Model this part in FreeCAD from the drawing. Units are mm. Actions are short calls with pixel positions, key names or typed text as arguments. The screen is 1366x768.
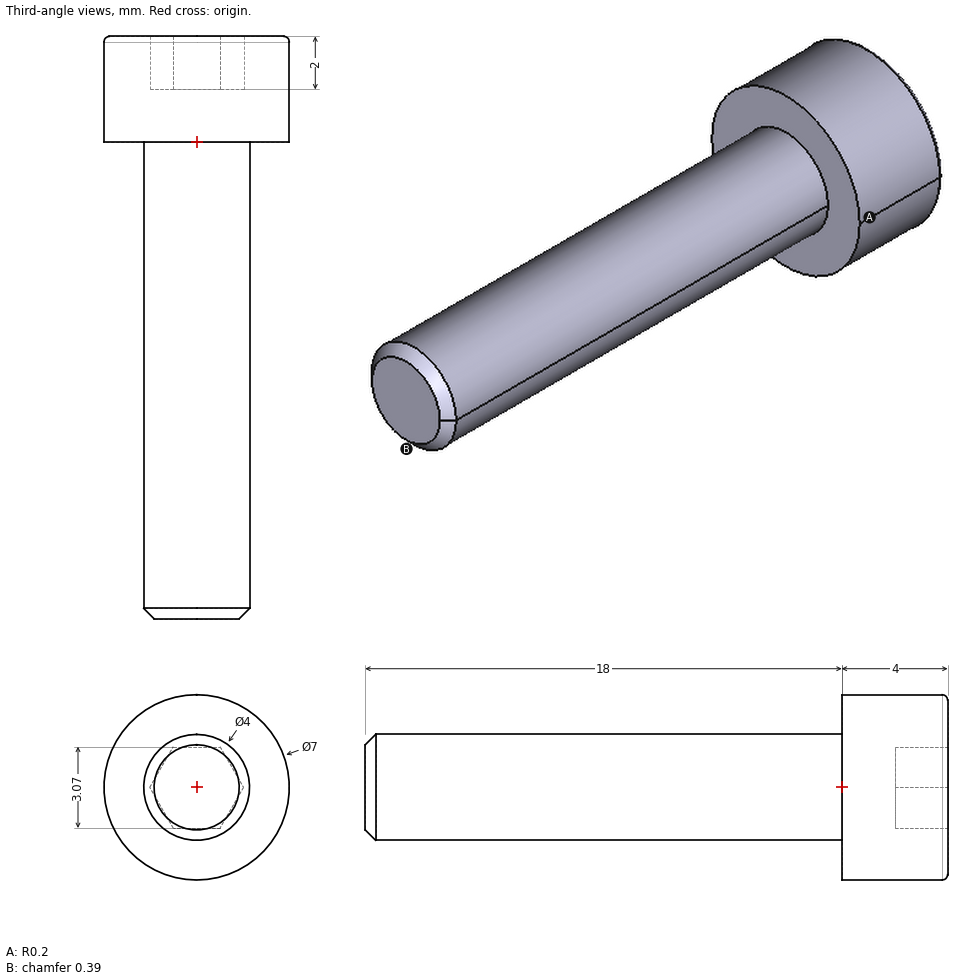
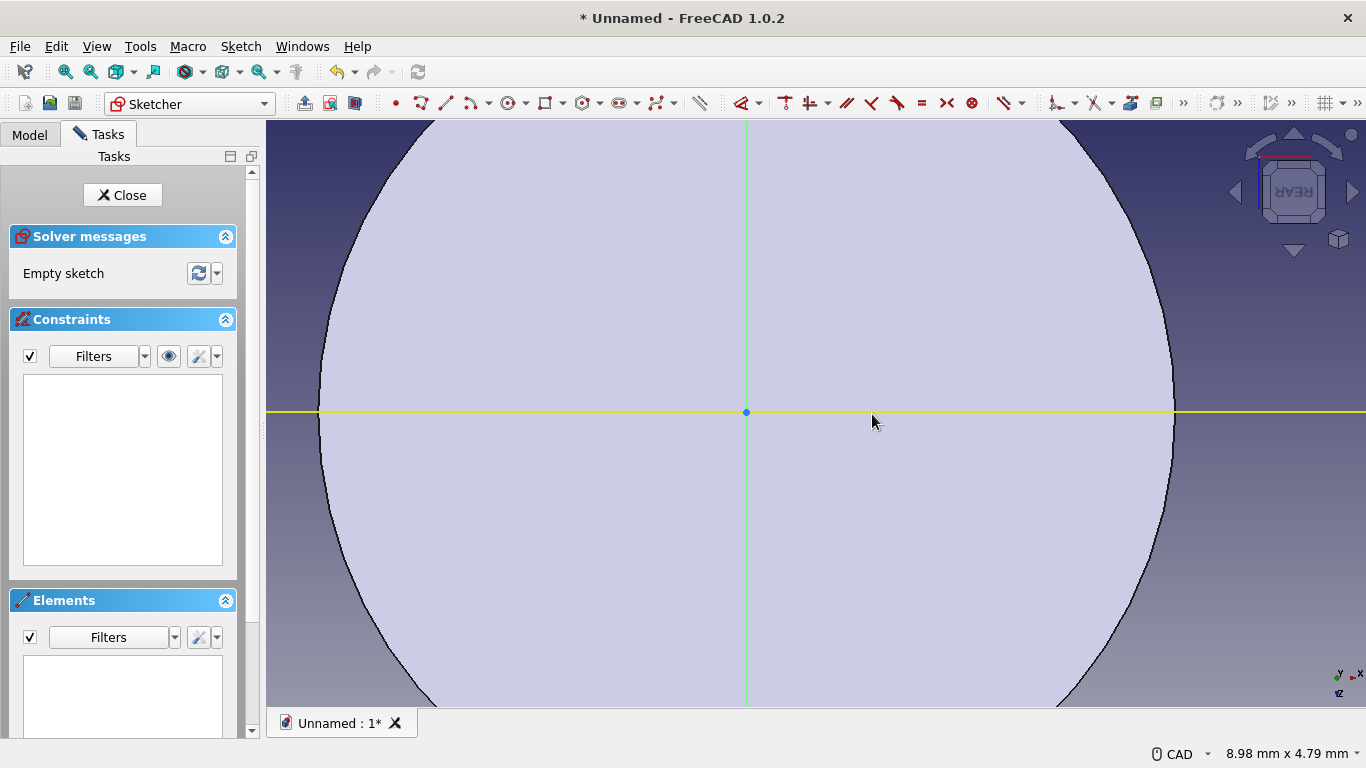
click(582, 104)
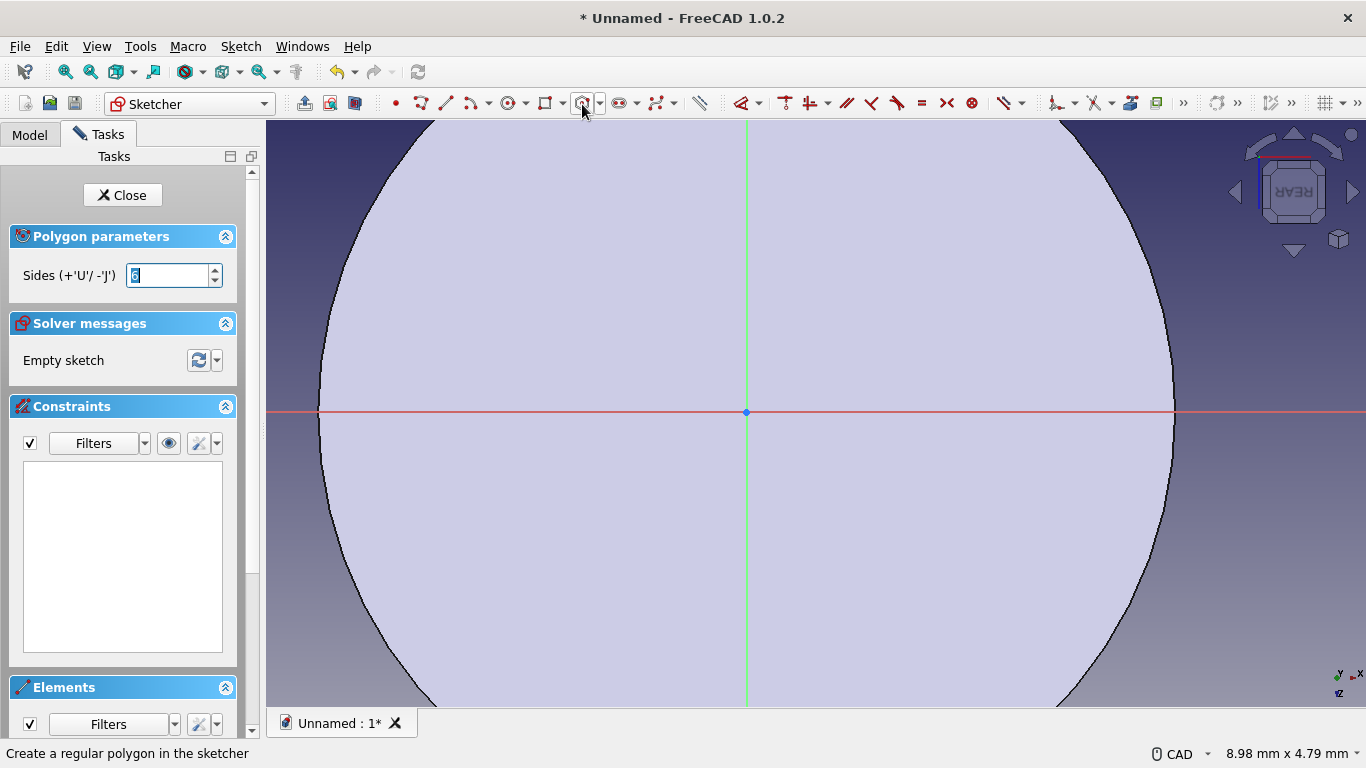
click(747, 412)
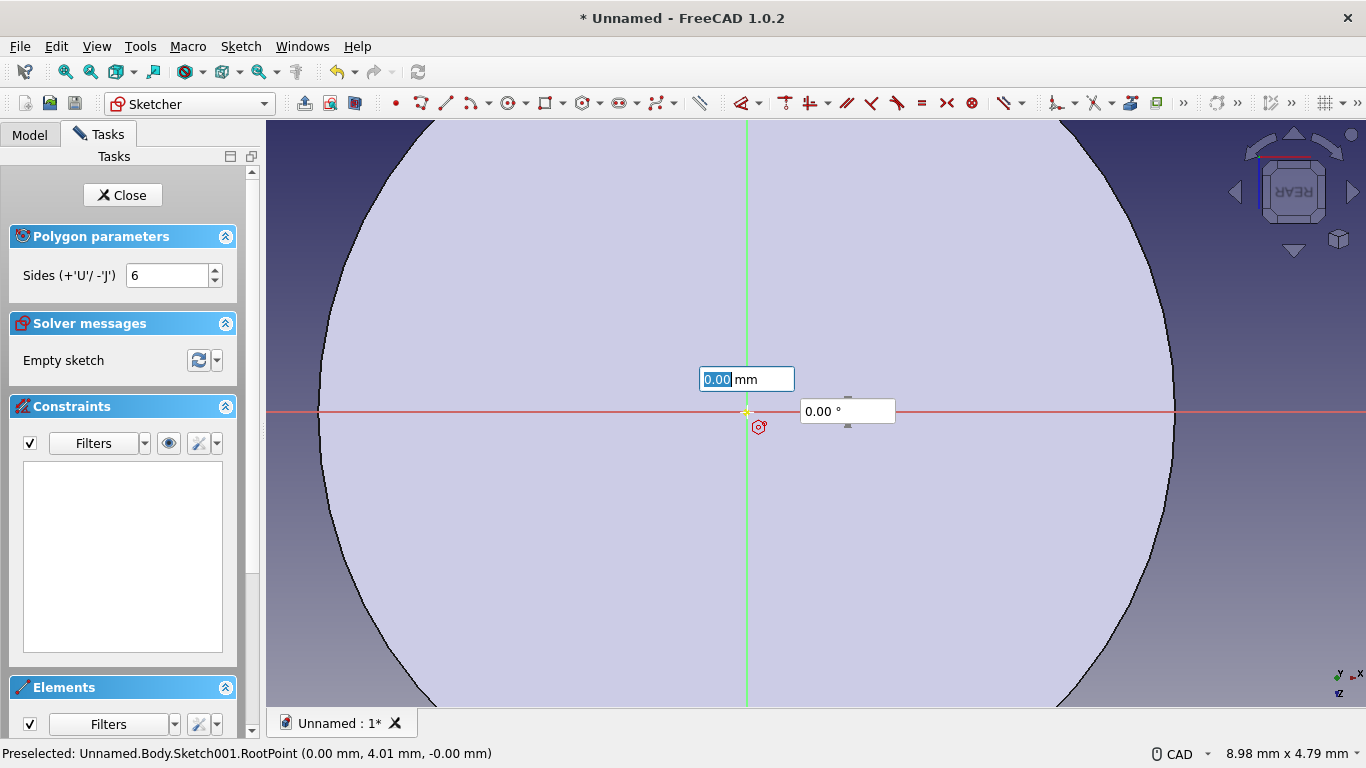
click(964, 412)
right_click(964, 412)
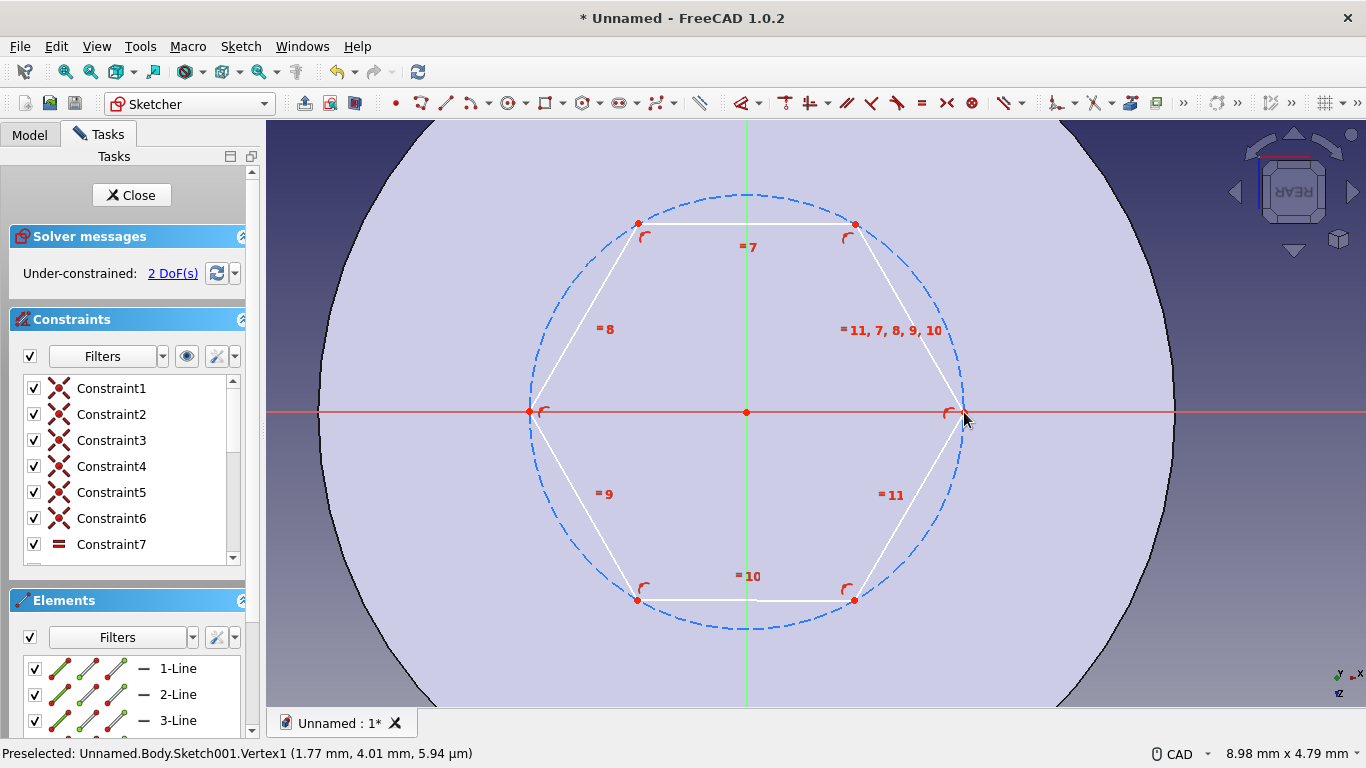
click(791, 224)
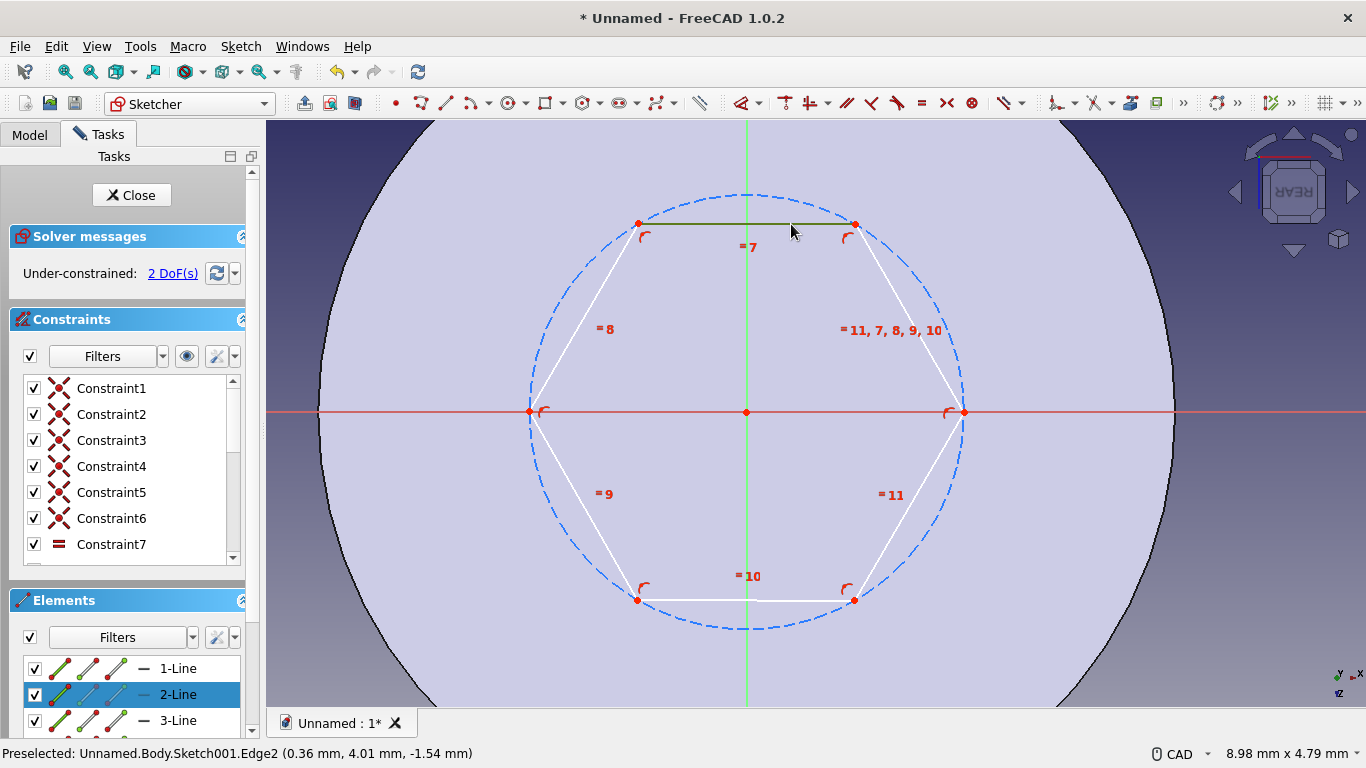
click(828, 104)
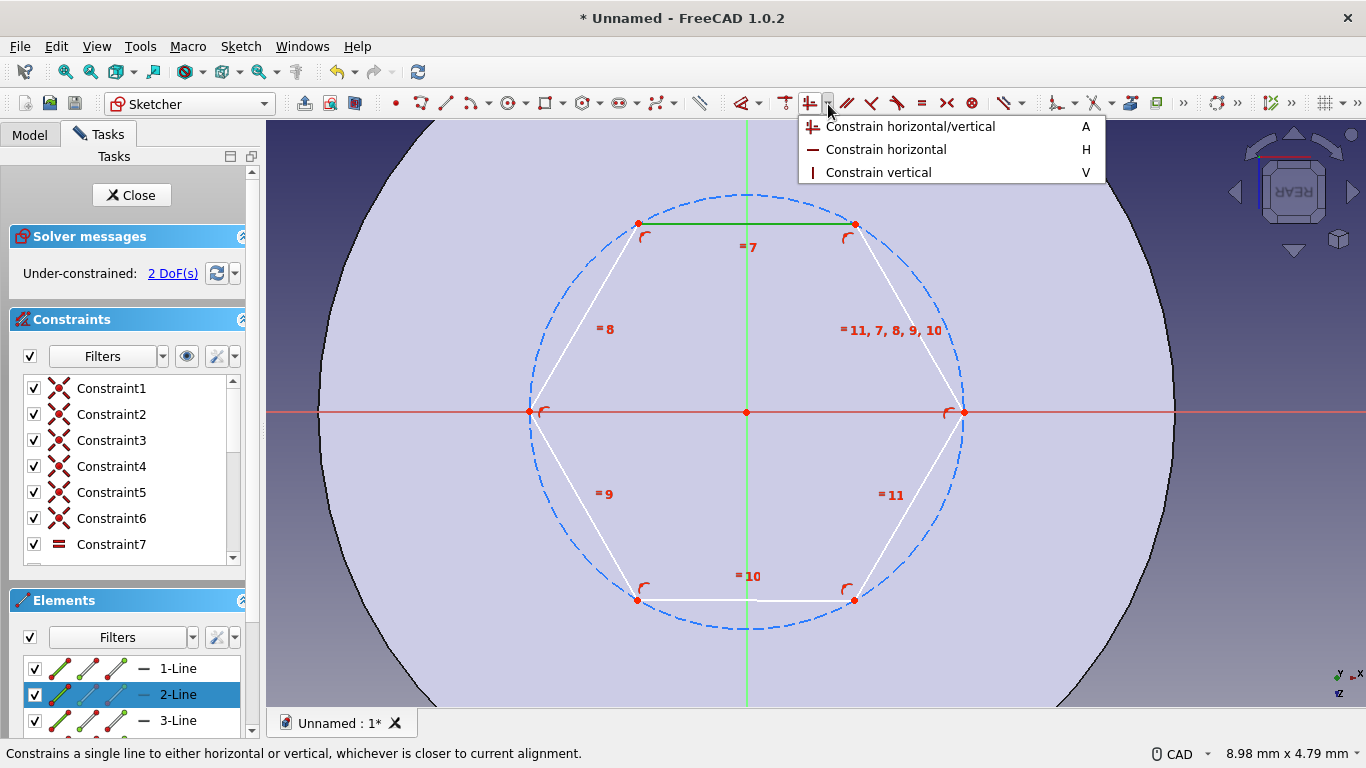
click(952, 150)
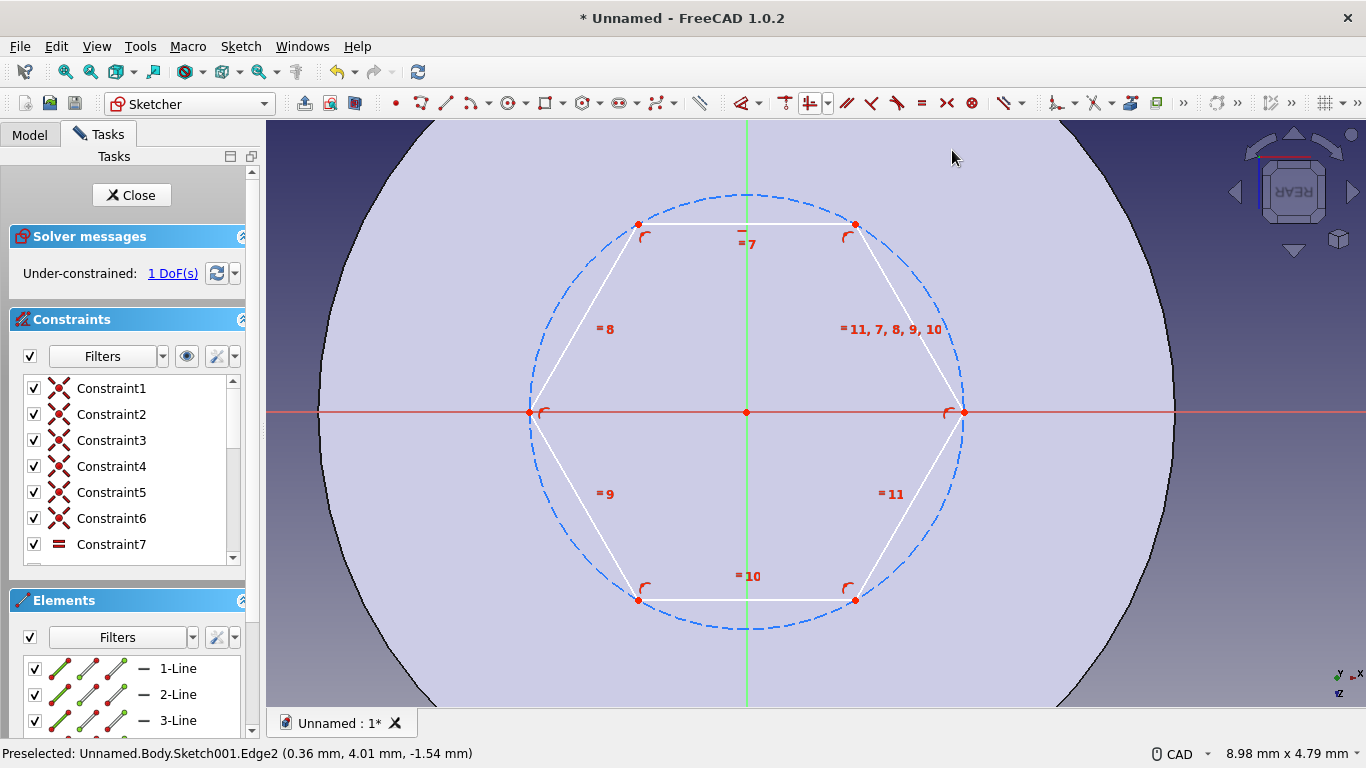
click(740, 104)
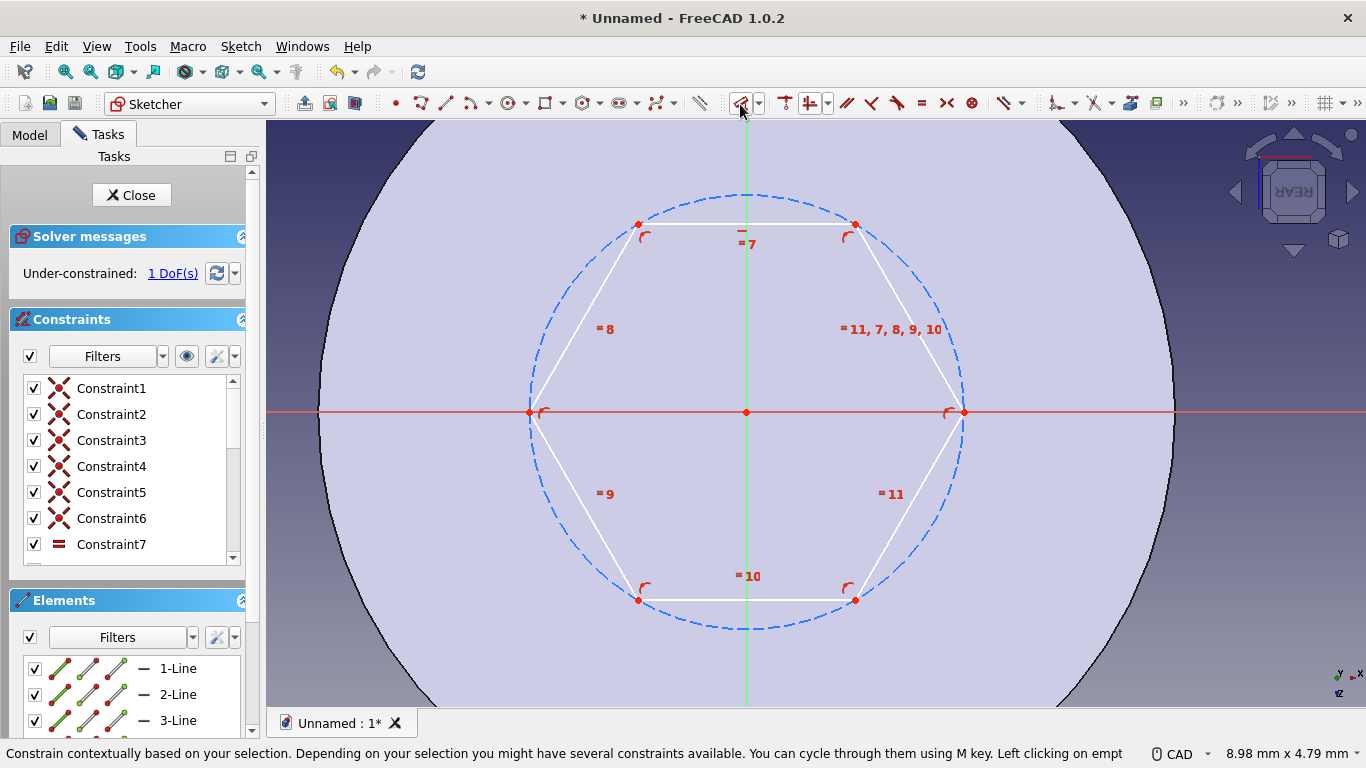
click(638, 600)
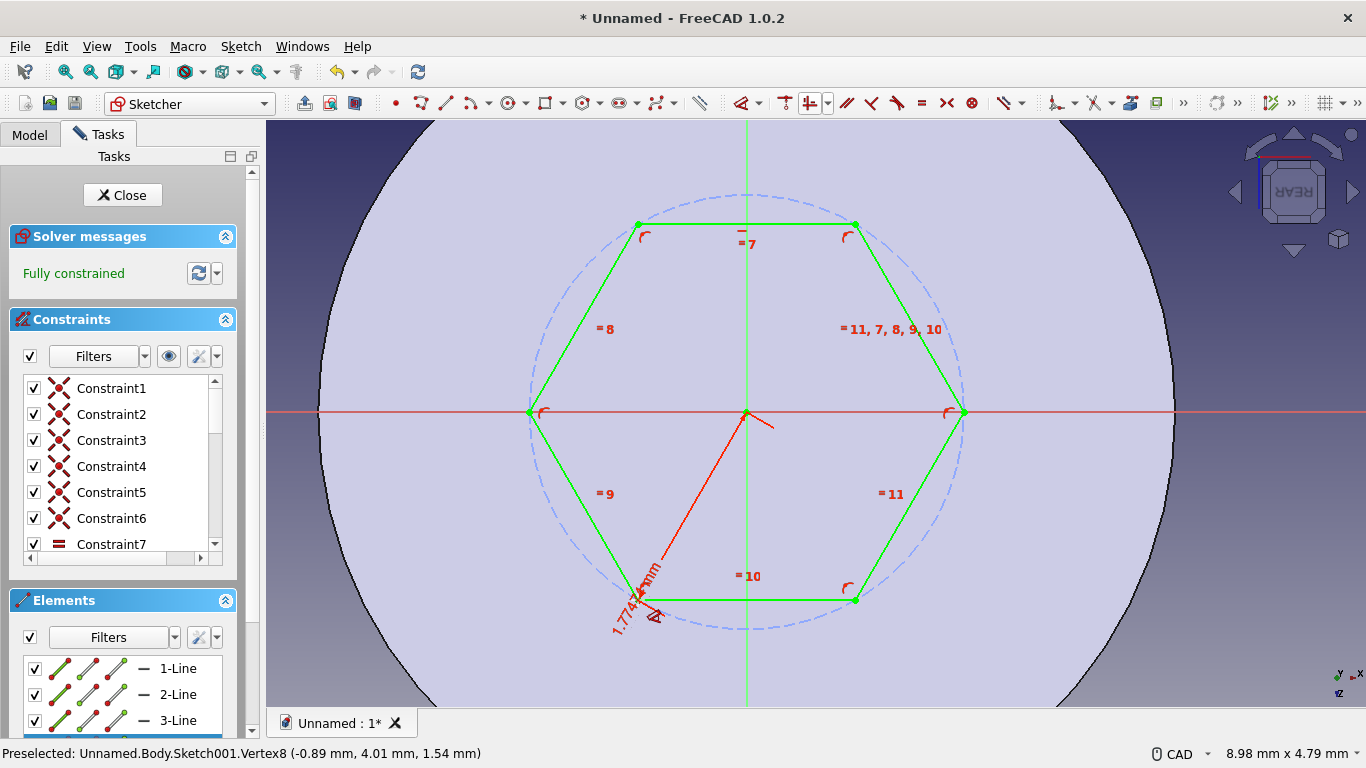
click(855, 224)
click(604, 326)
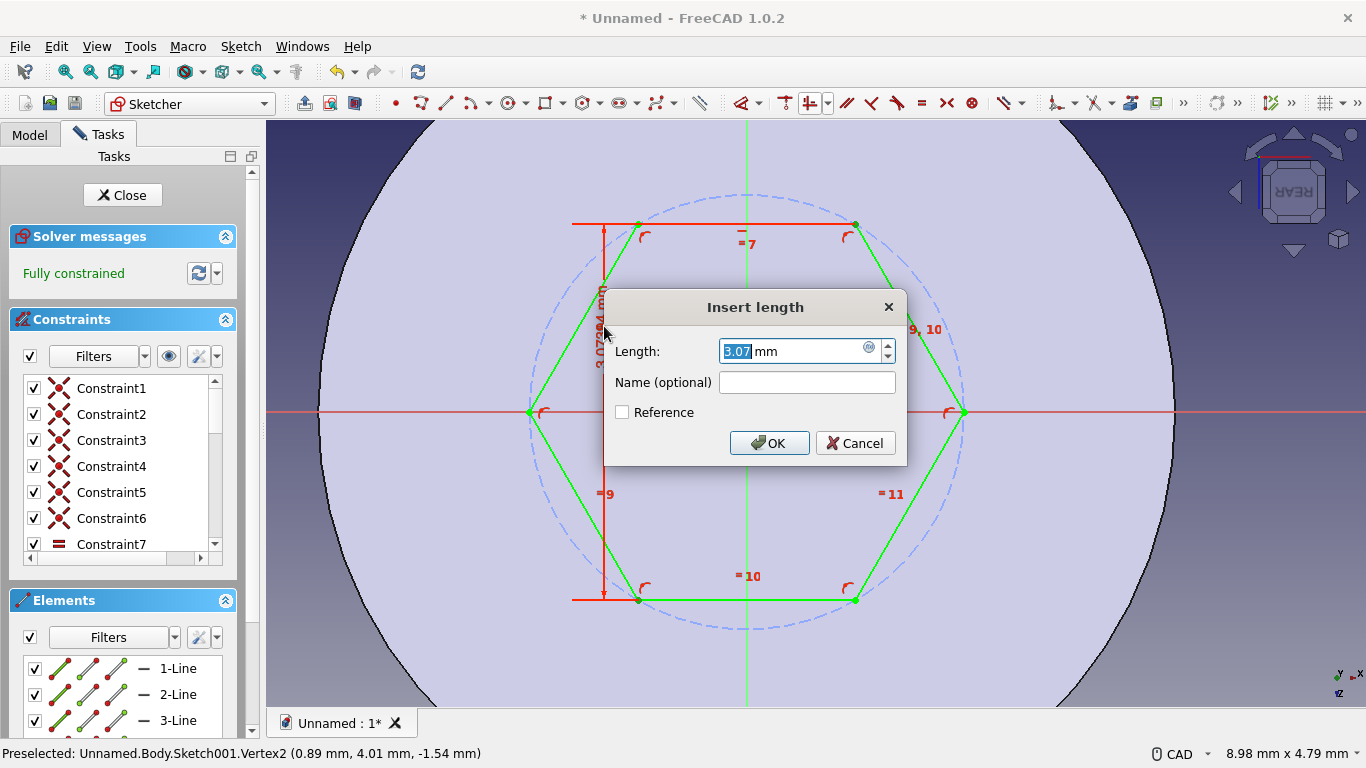
text(3.07)
key(Return)
key(Escape)